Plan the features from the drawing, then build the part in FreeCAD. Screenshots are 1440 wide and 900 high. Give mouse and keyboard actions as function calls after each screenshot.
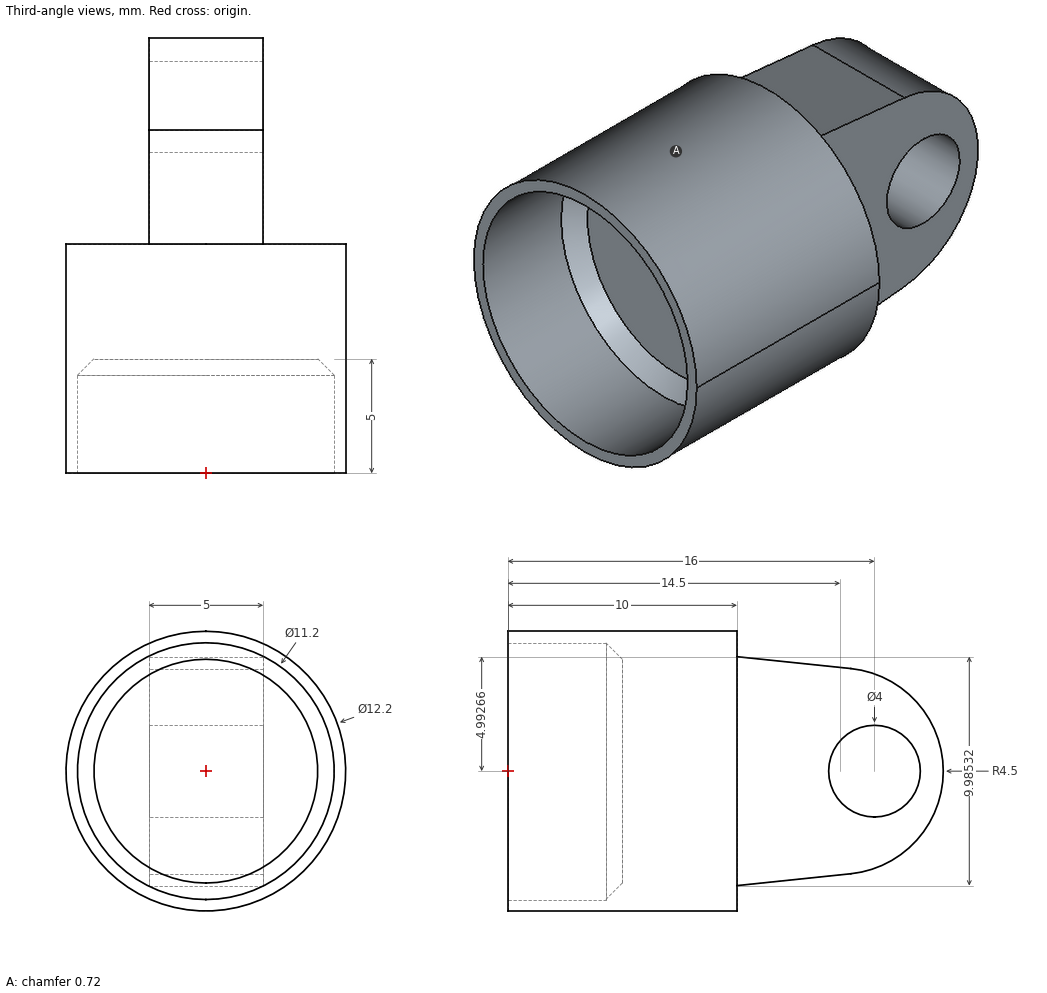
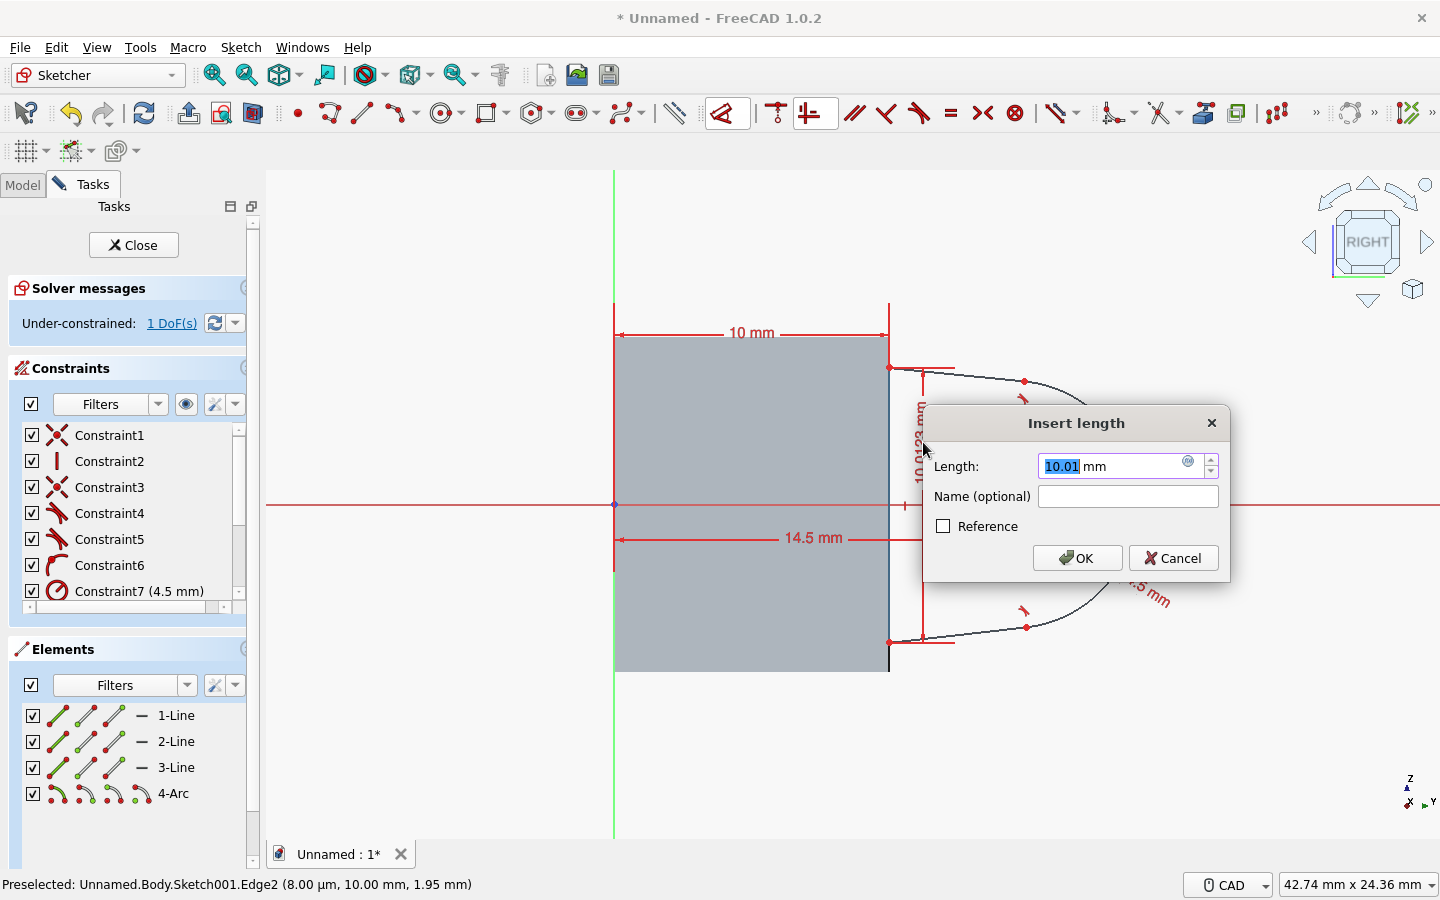
text(9.98532)
key(Return)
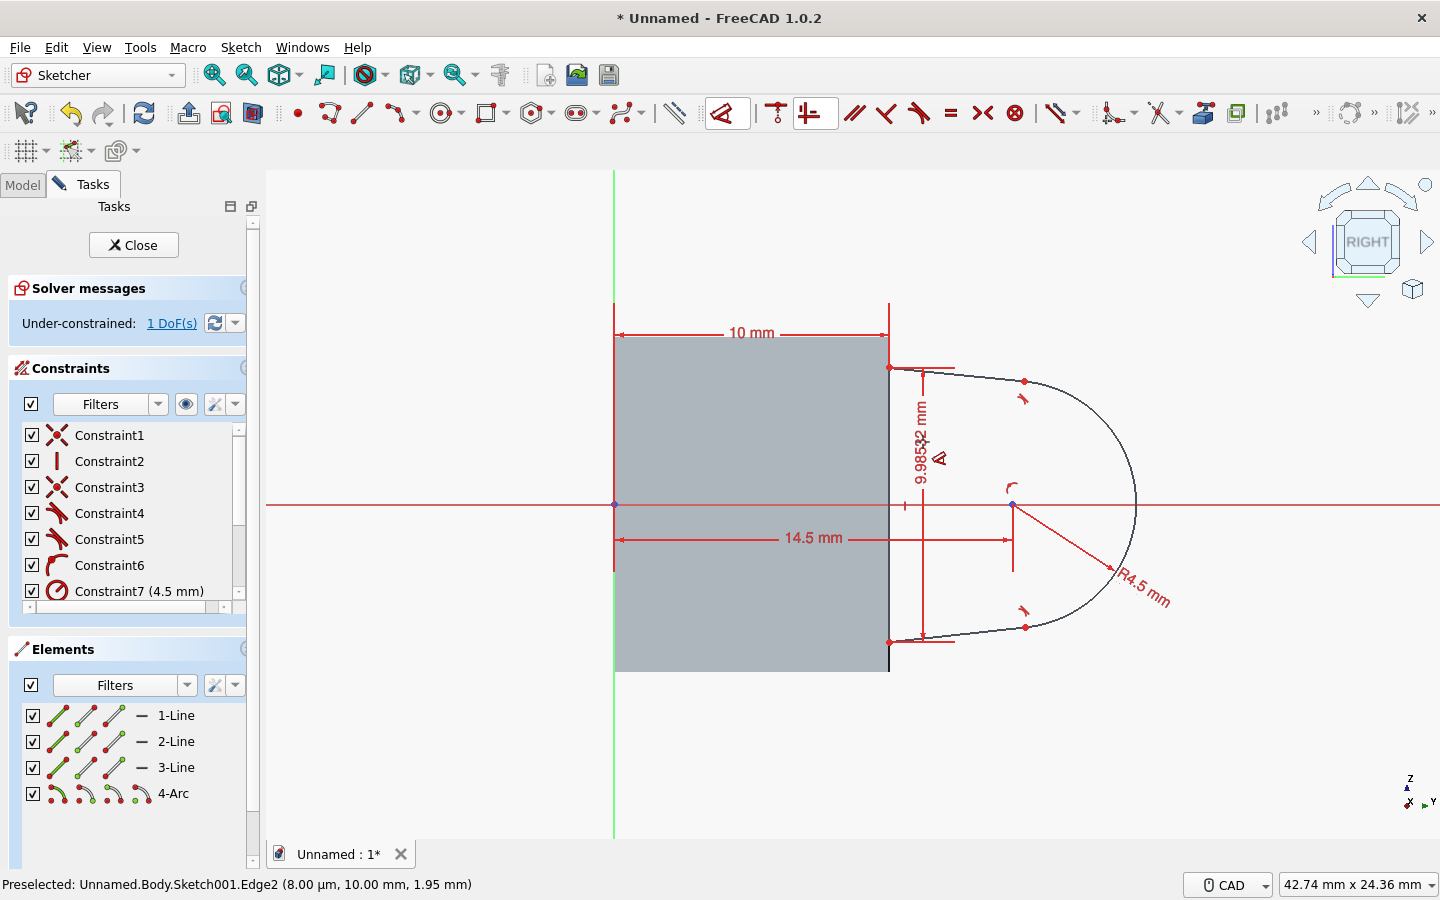
click(889, 368)
click(580, 436)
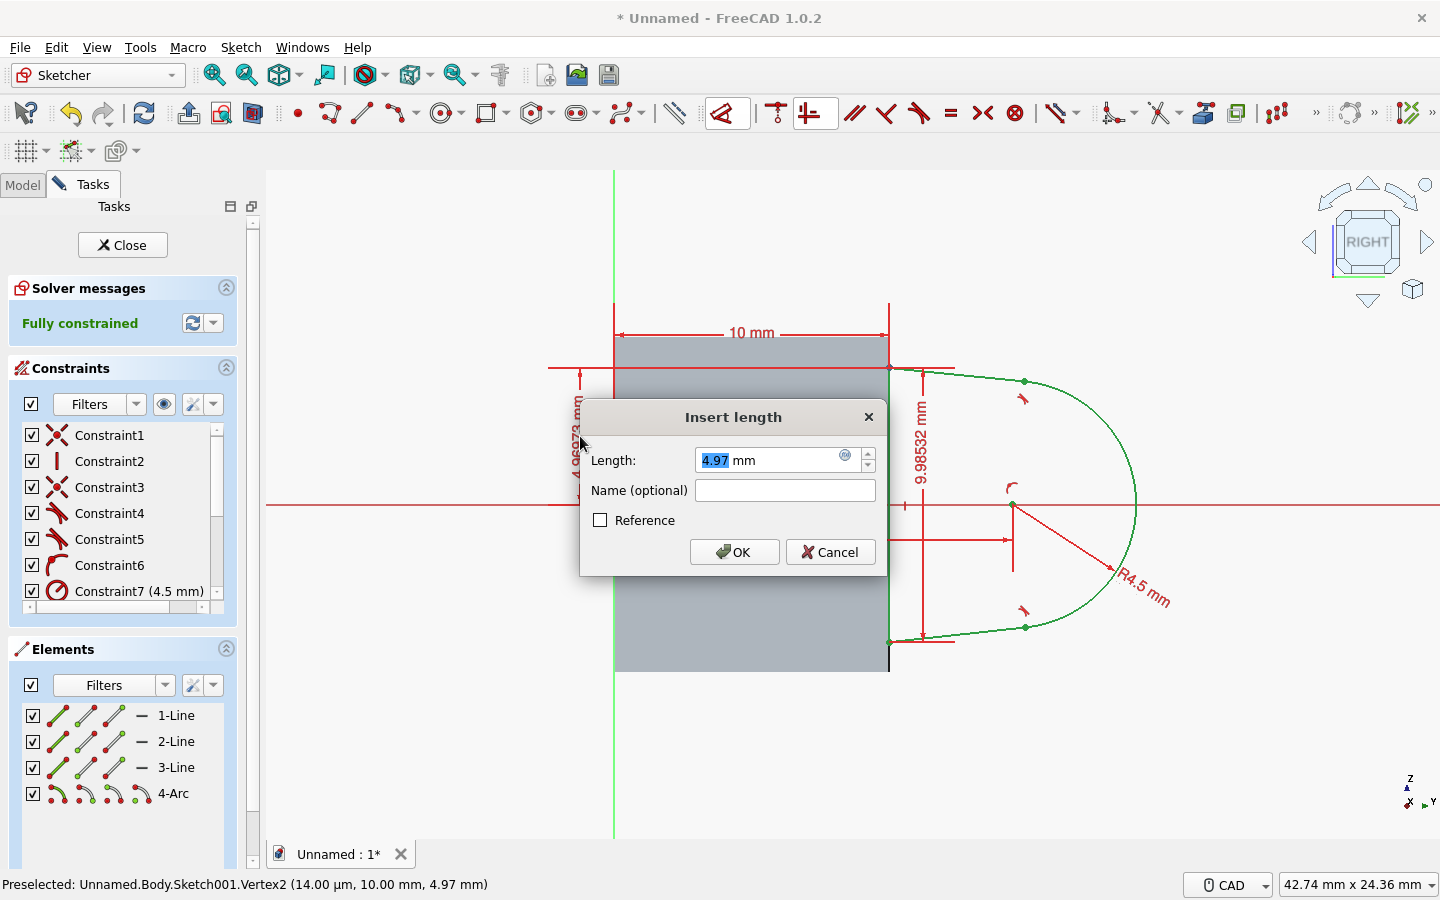
text(4.99266)
key(Return)
key(Escape)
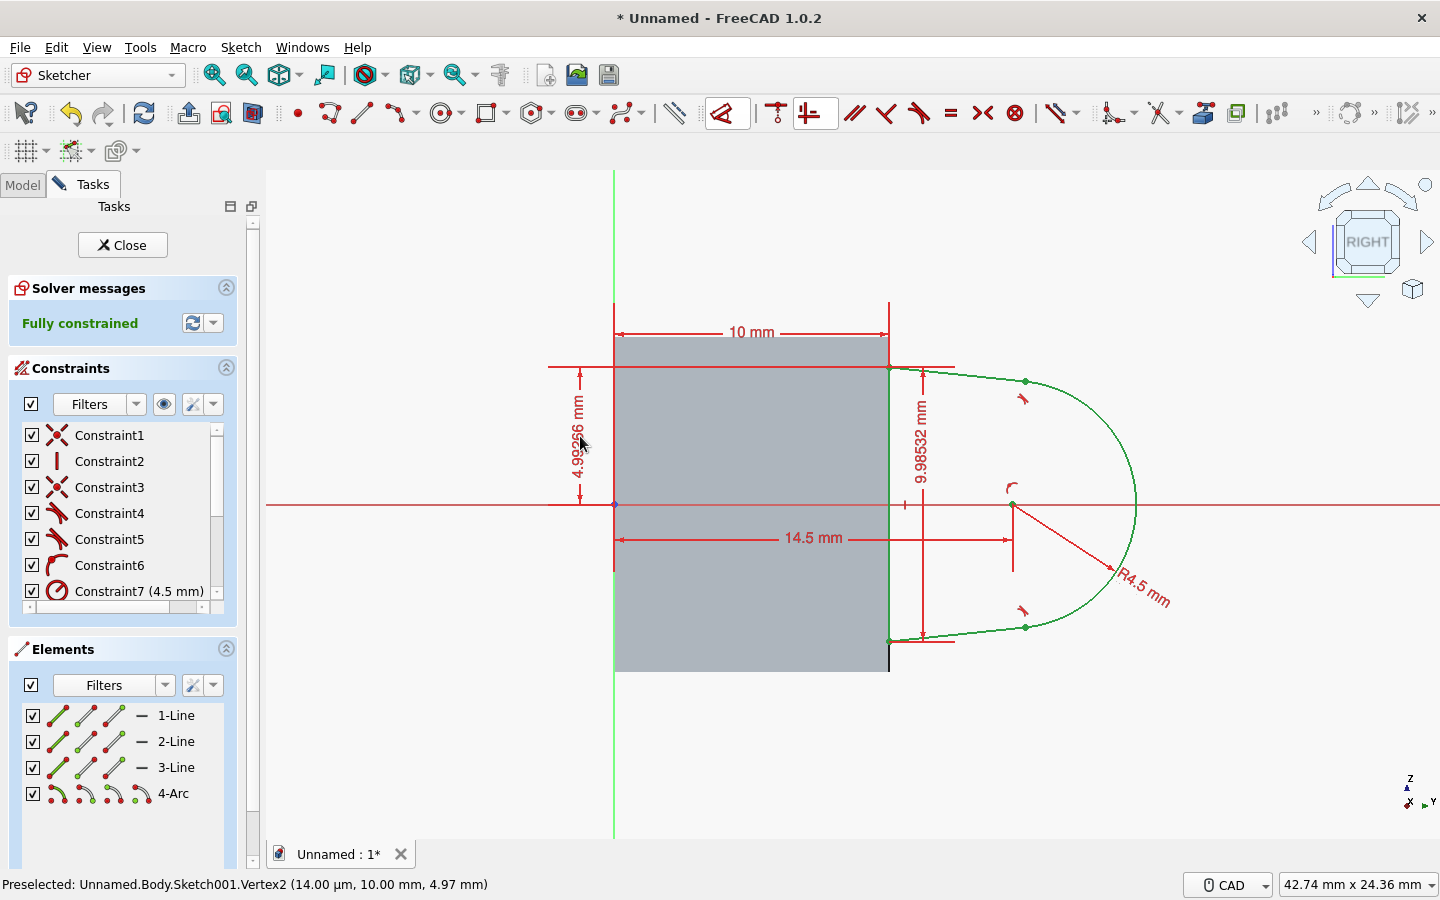
click(123, 245)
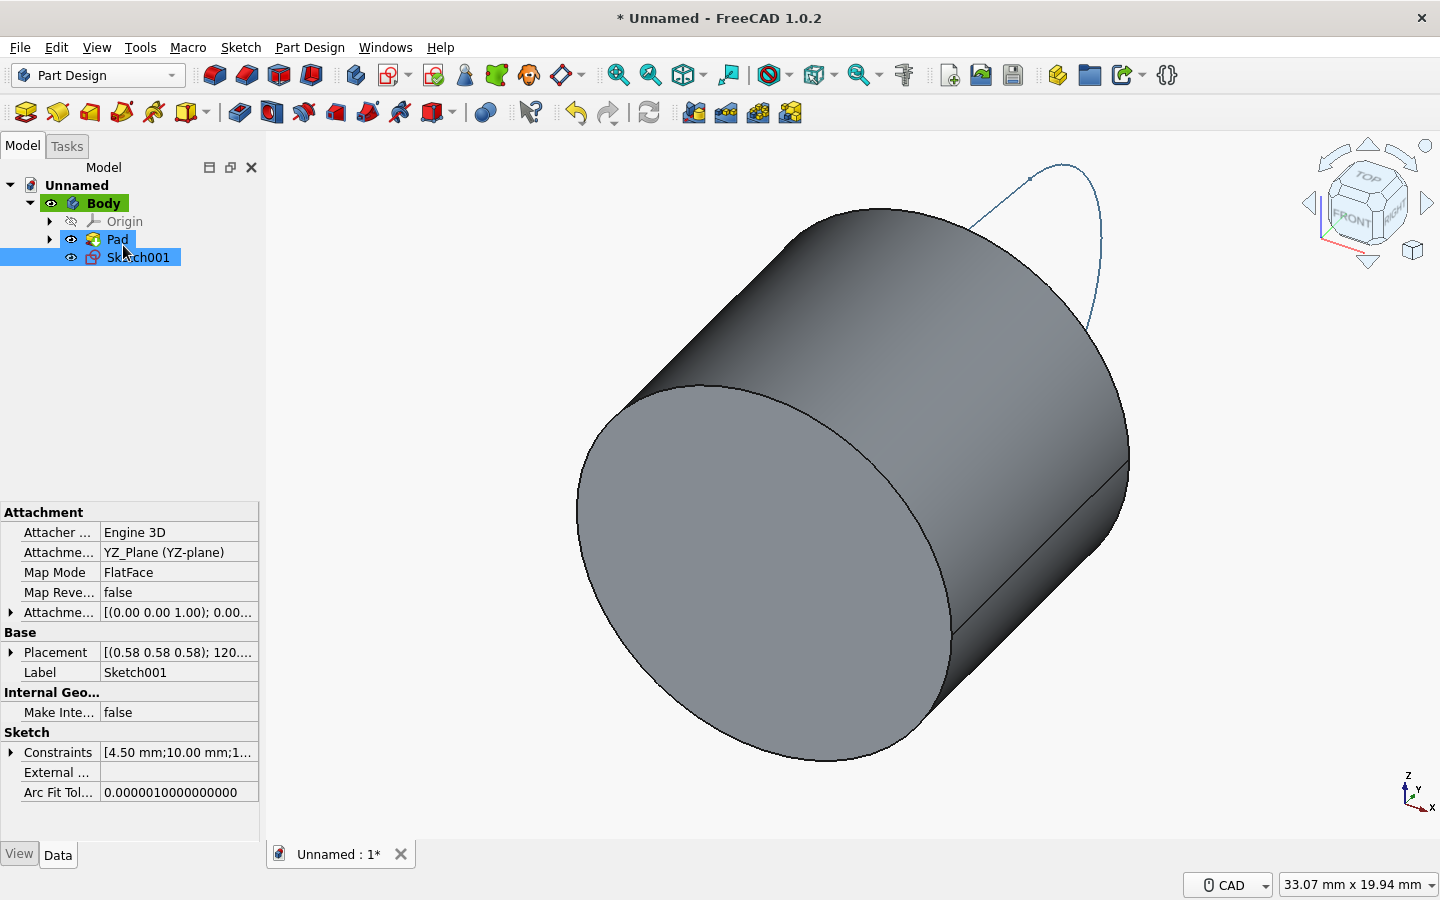
click(26, 112)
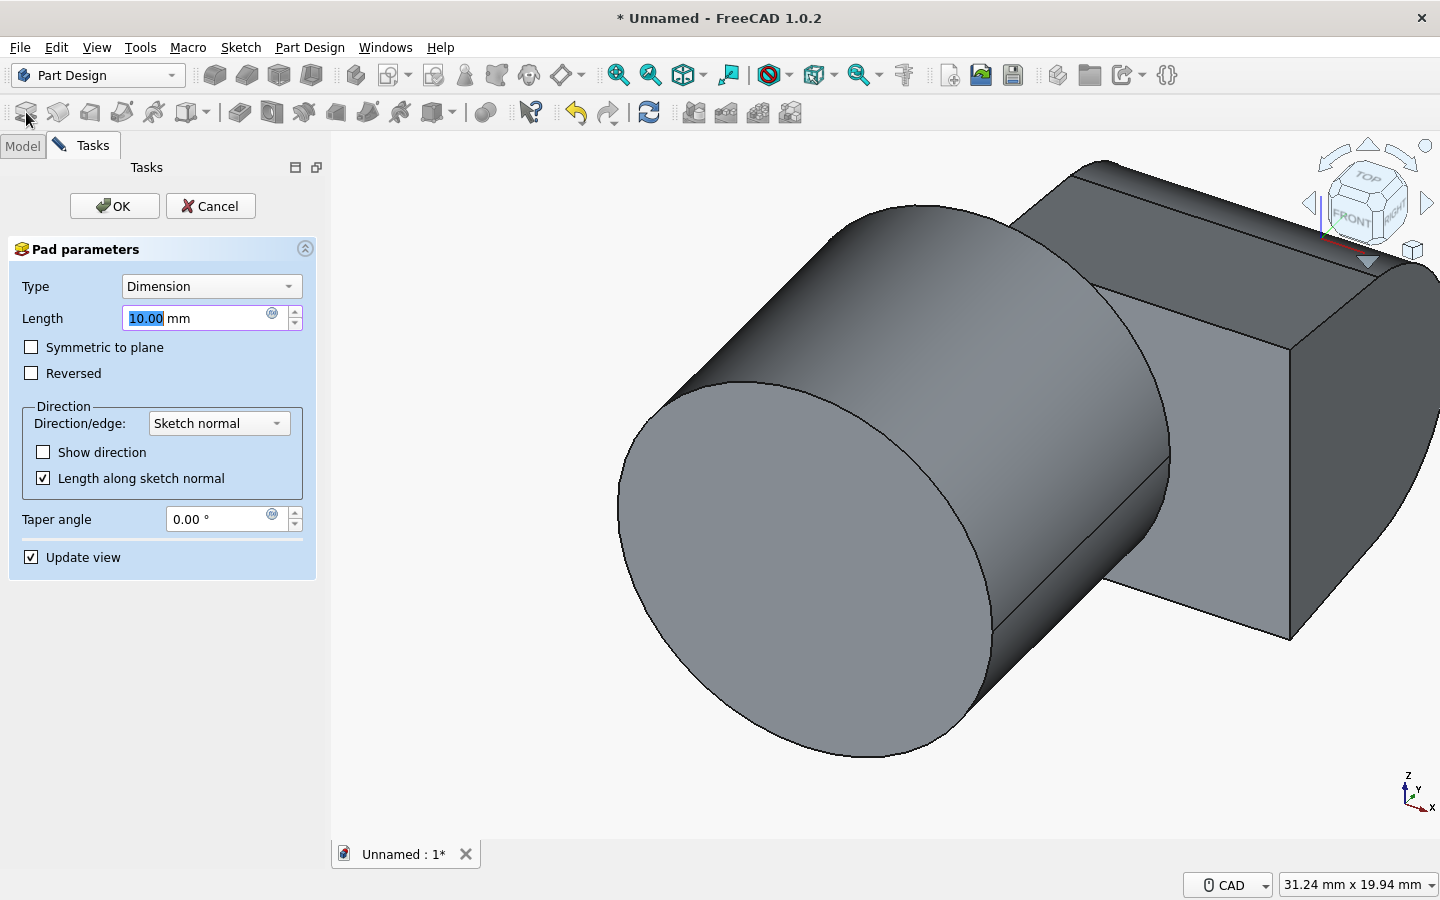
text(5)
key(Tab)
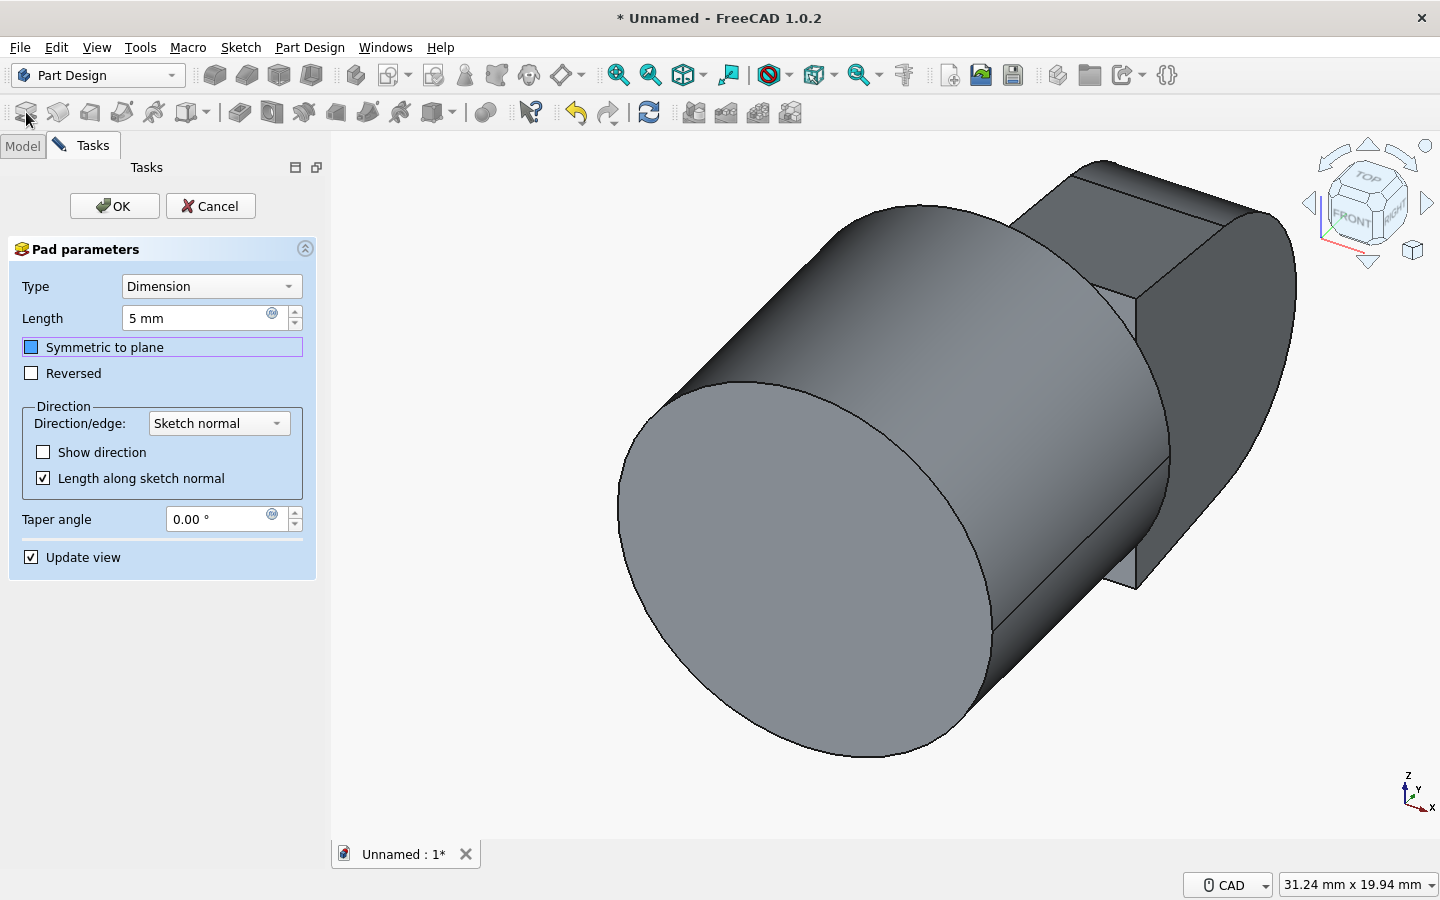
click(30, 347)